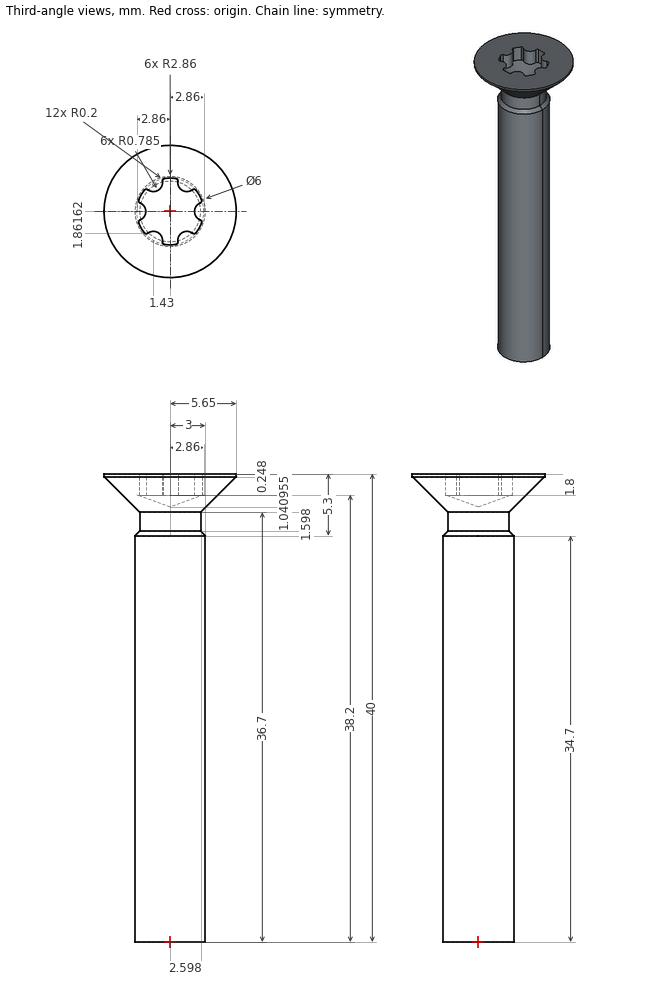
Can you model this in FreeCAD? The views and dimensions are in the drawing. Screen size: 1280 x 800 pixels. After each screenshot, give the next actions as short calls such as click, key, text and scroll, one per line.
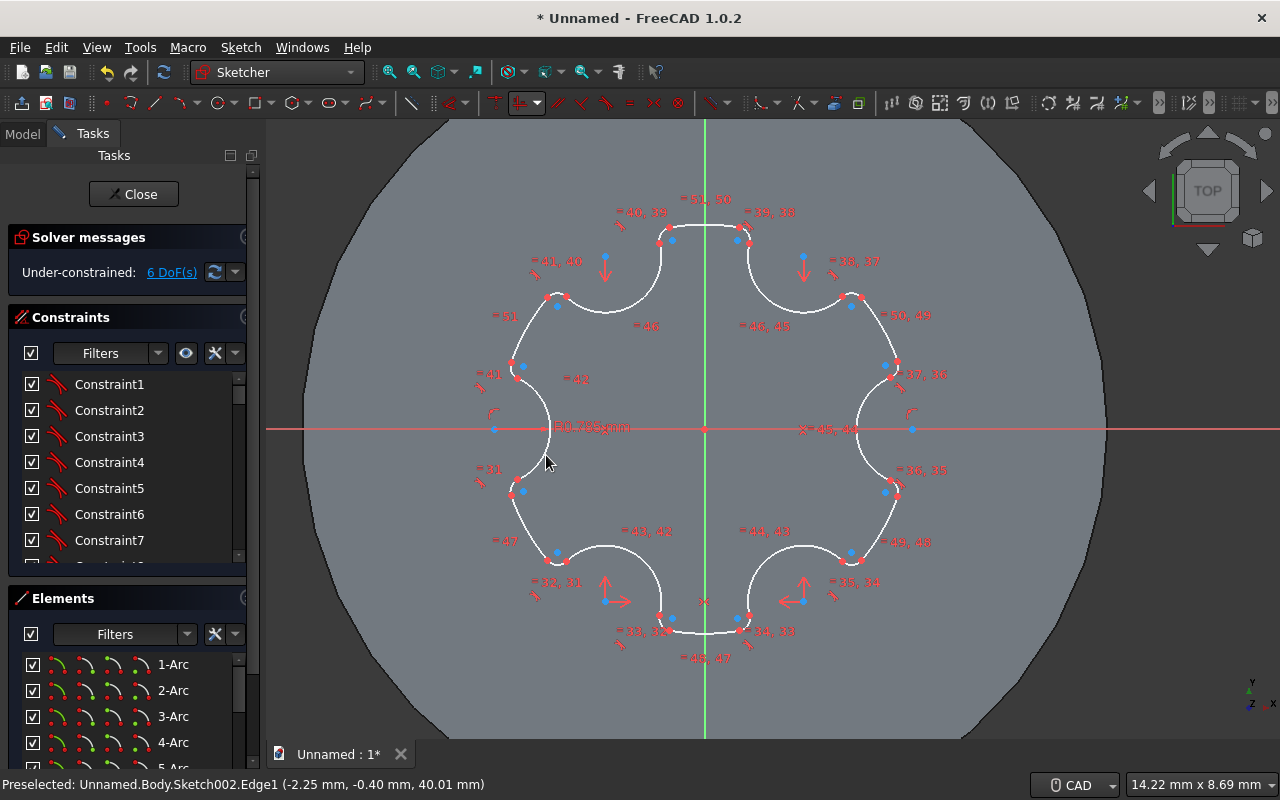
scroll(512, 486, up, 6)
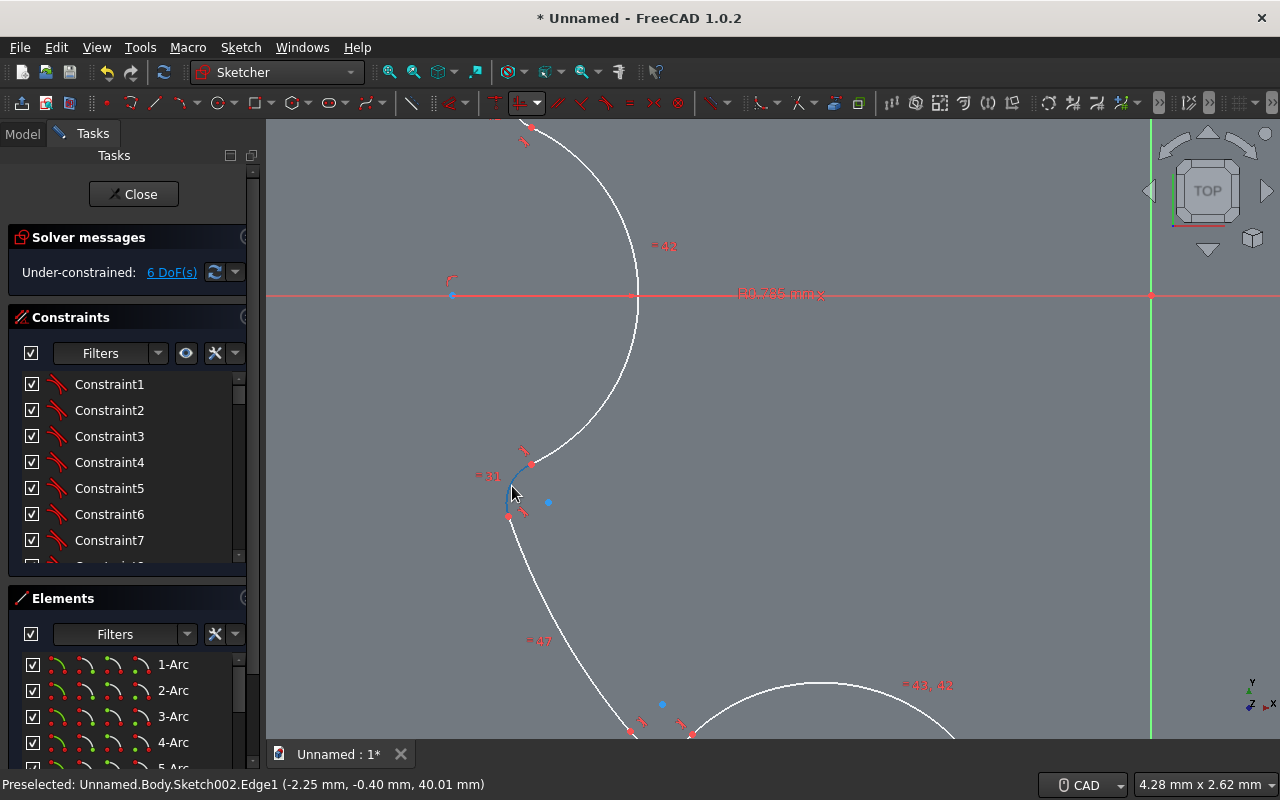
click(510, 486)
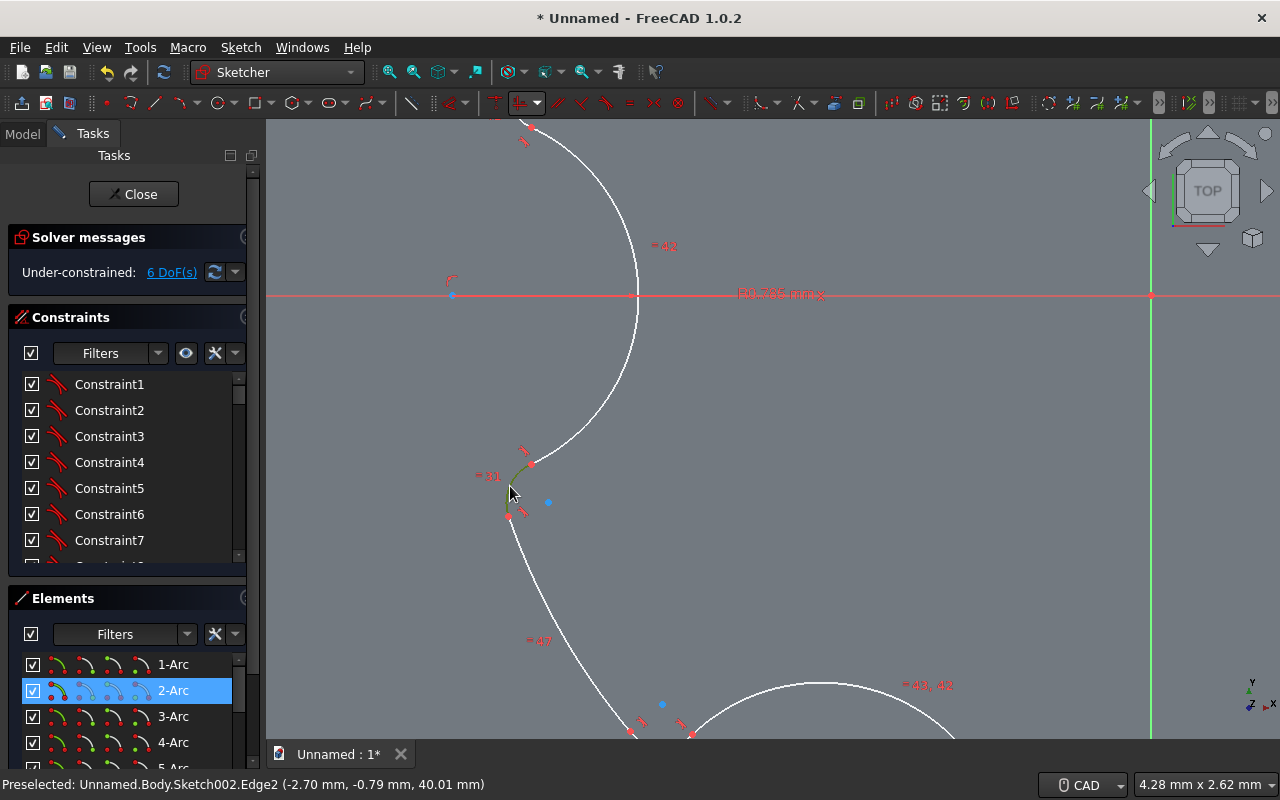
key(k)
key(r)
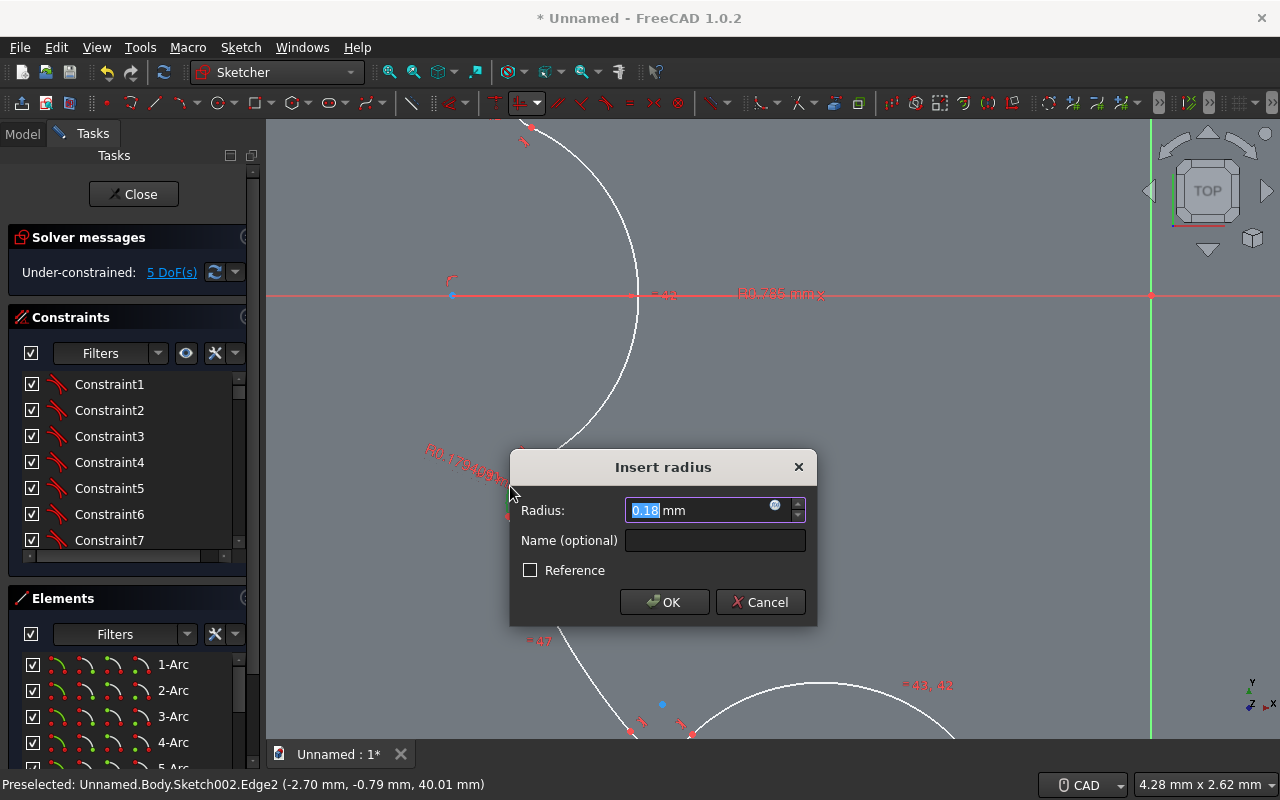
text(0.2)
key(Return)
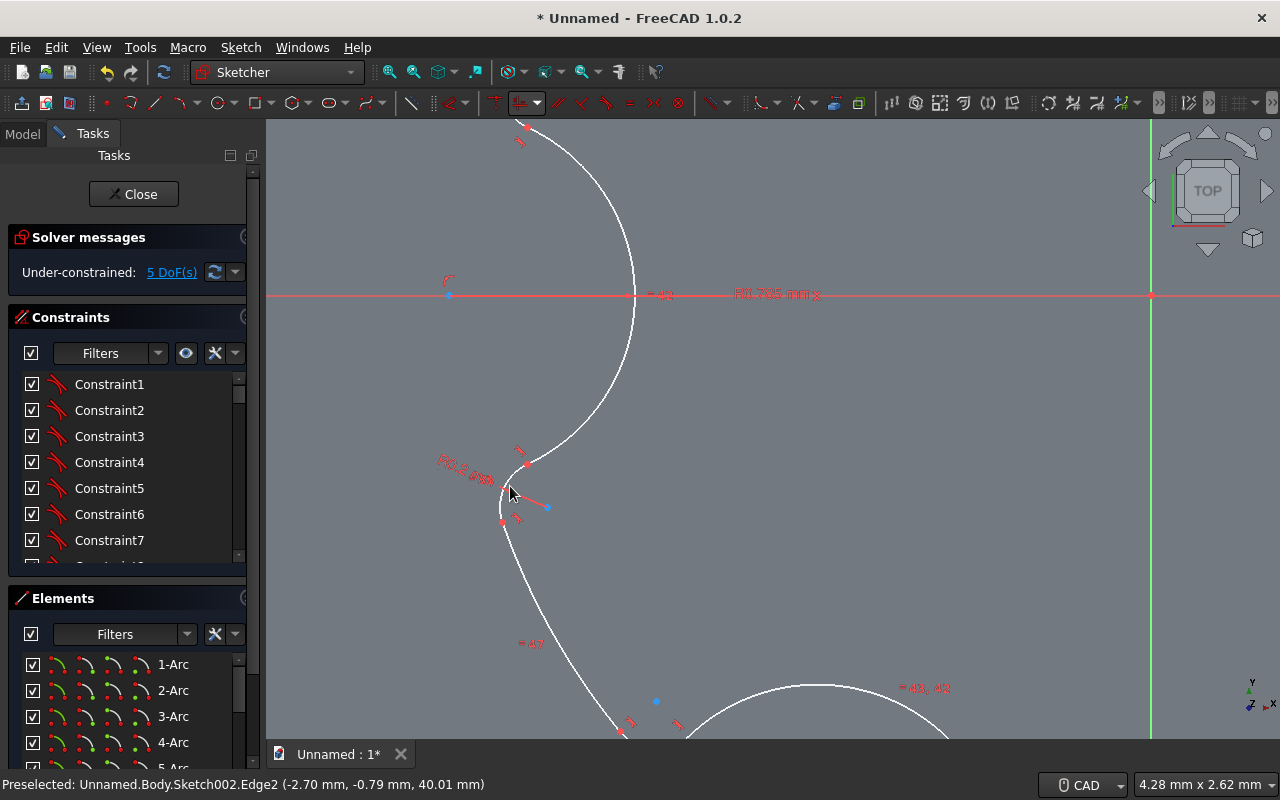
click(530, 590)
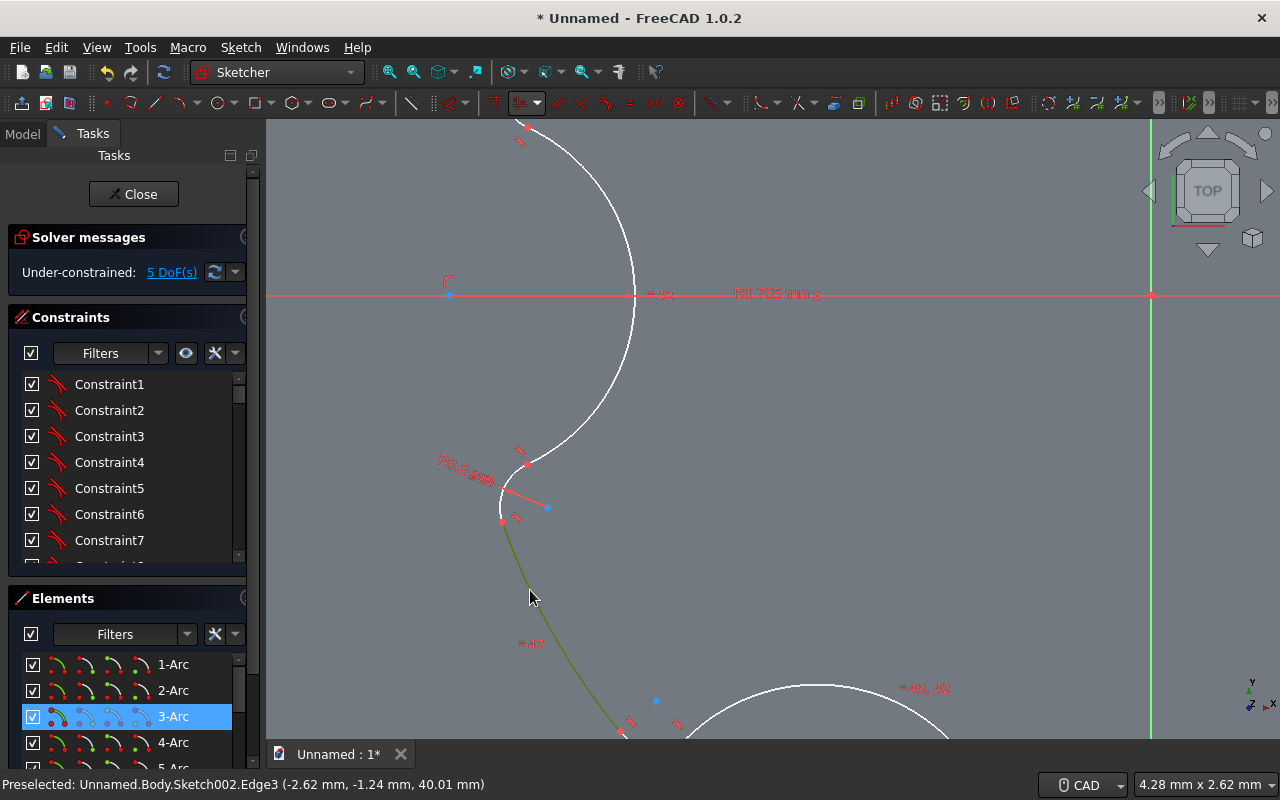
click(468, 104)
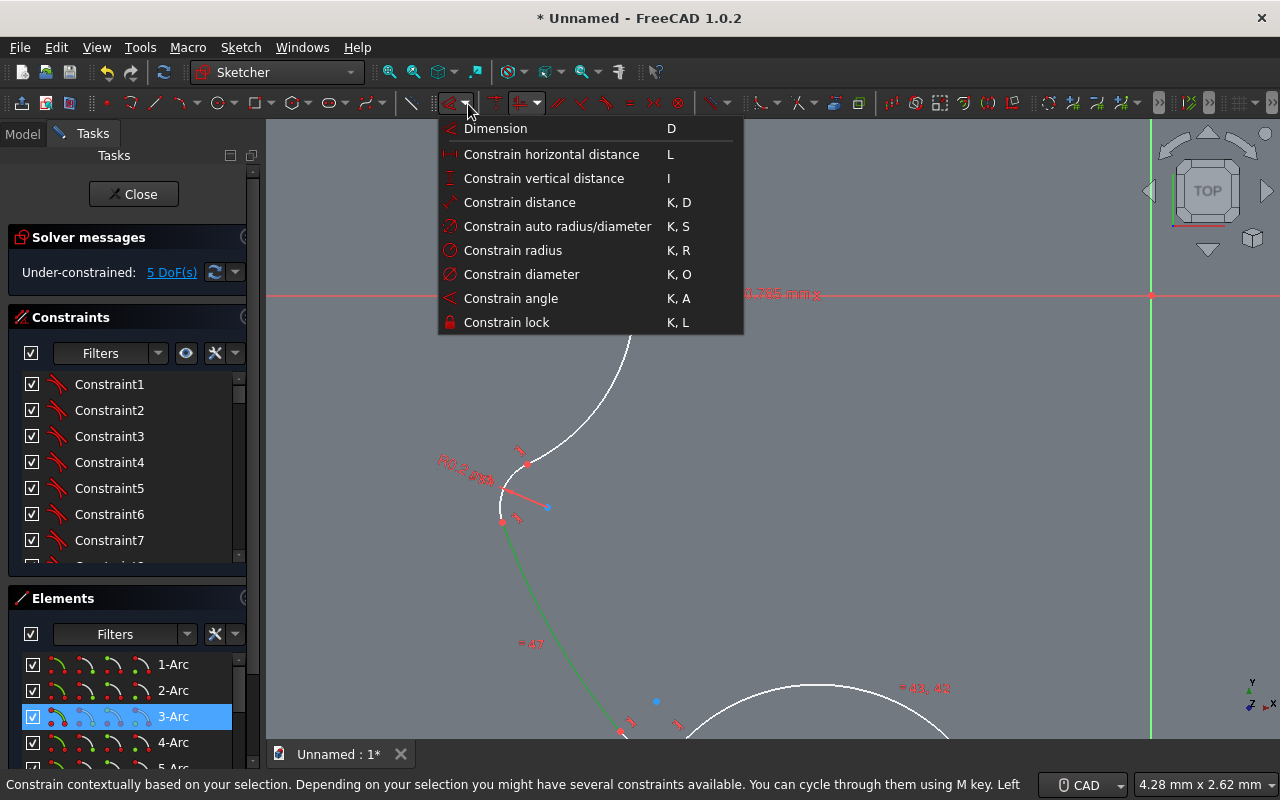
click(591, 250)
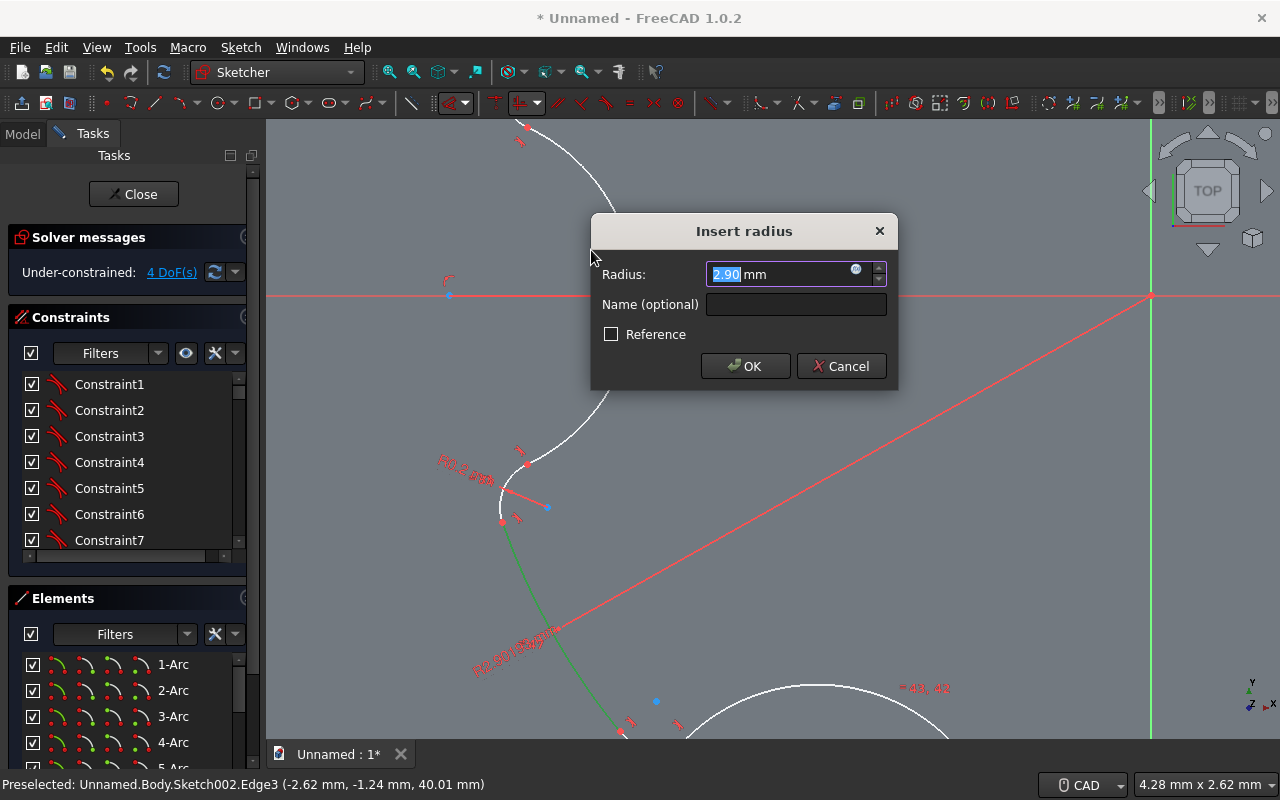
text(2.86)
key(Return)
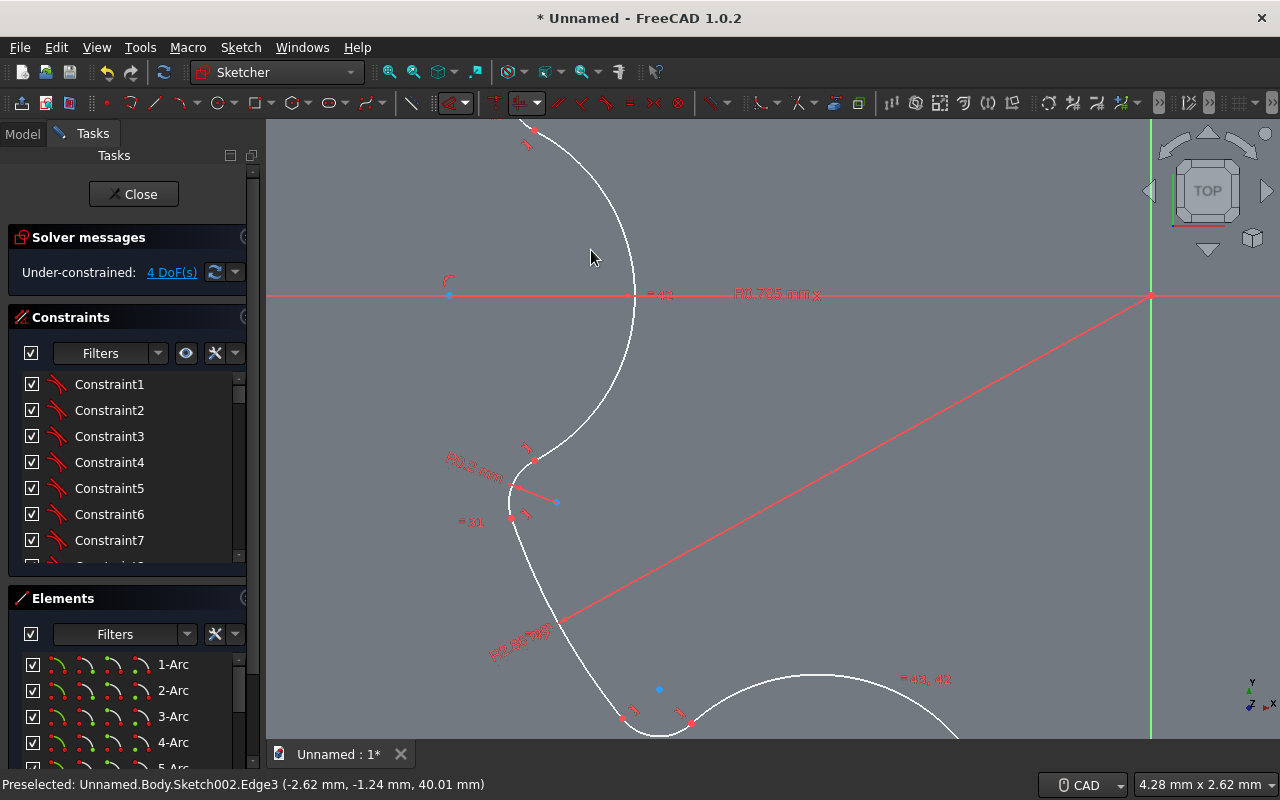
click(449, 296)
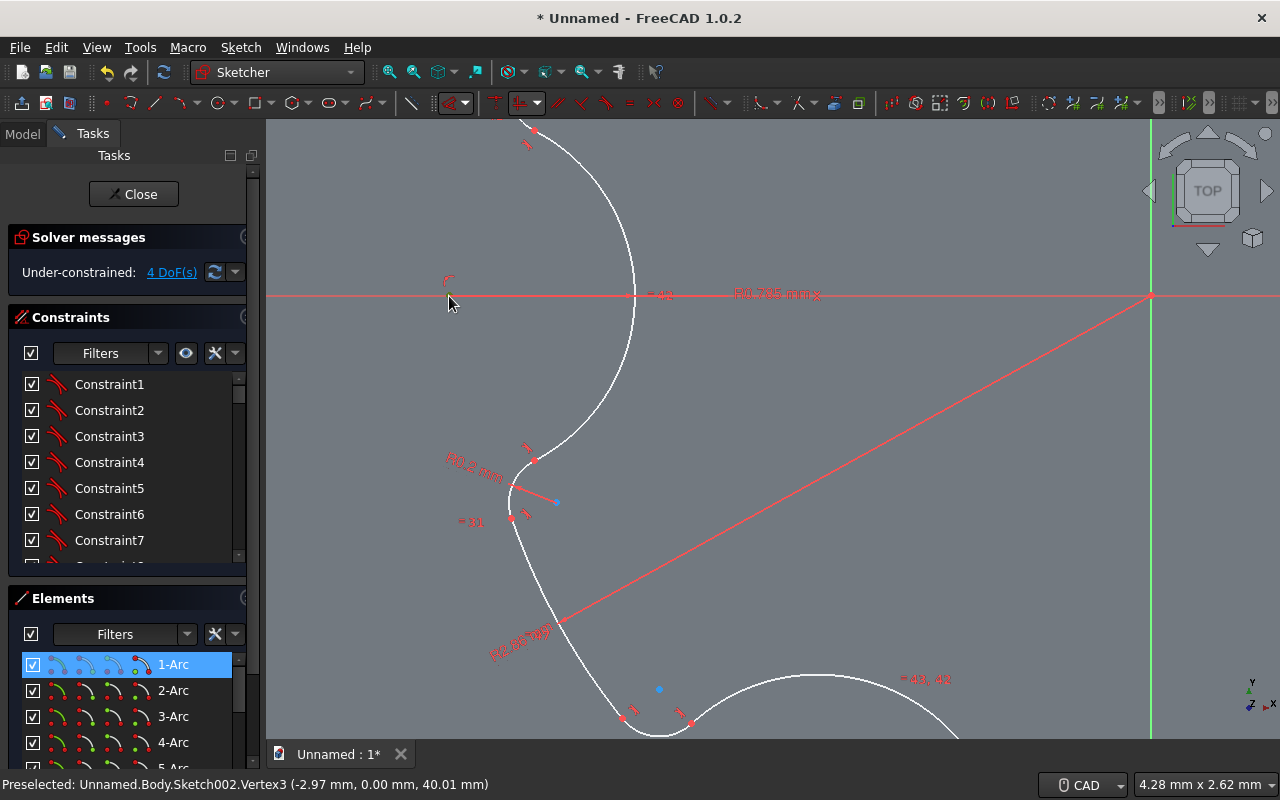
click(468, 104)